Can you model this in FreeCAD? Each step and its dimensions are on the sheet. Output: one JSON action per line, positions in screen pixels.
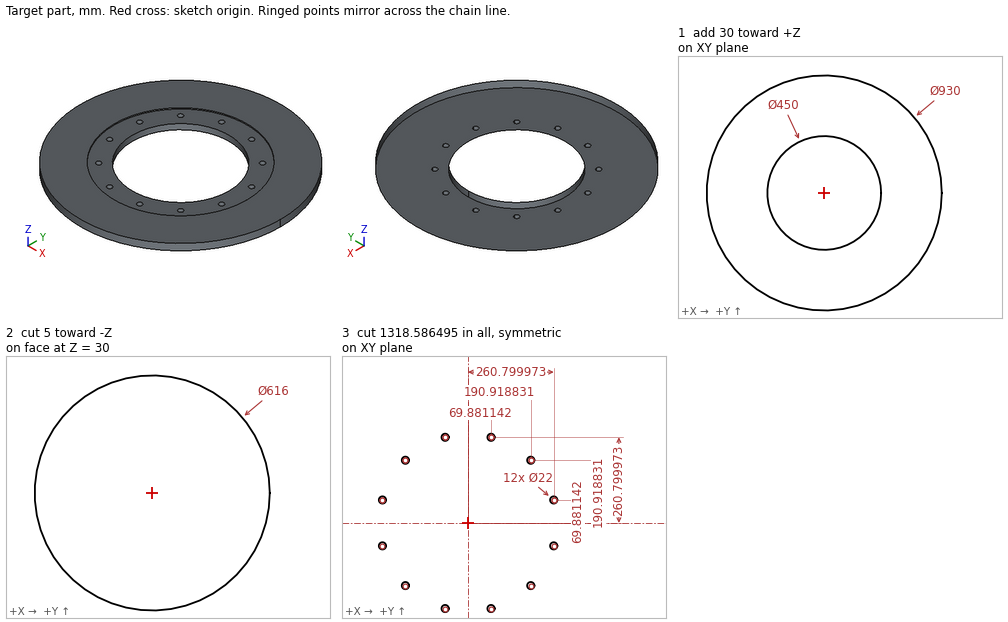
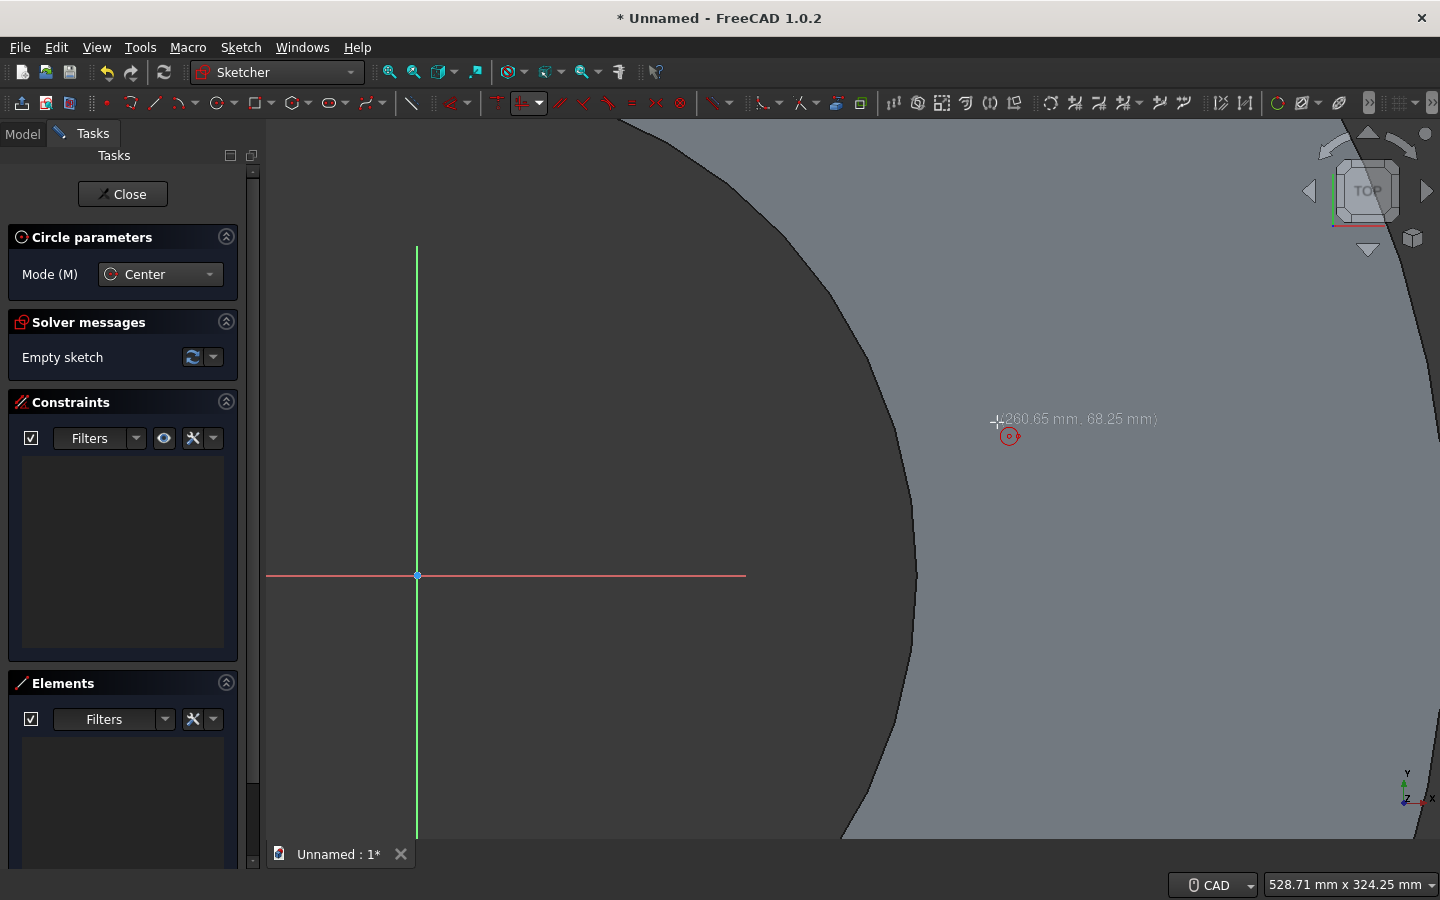
{"action": "left_click", "coordinate": [996, 420]}
{"action": "mouse_move", "coordinate": [1014, 403]}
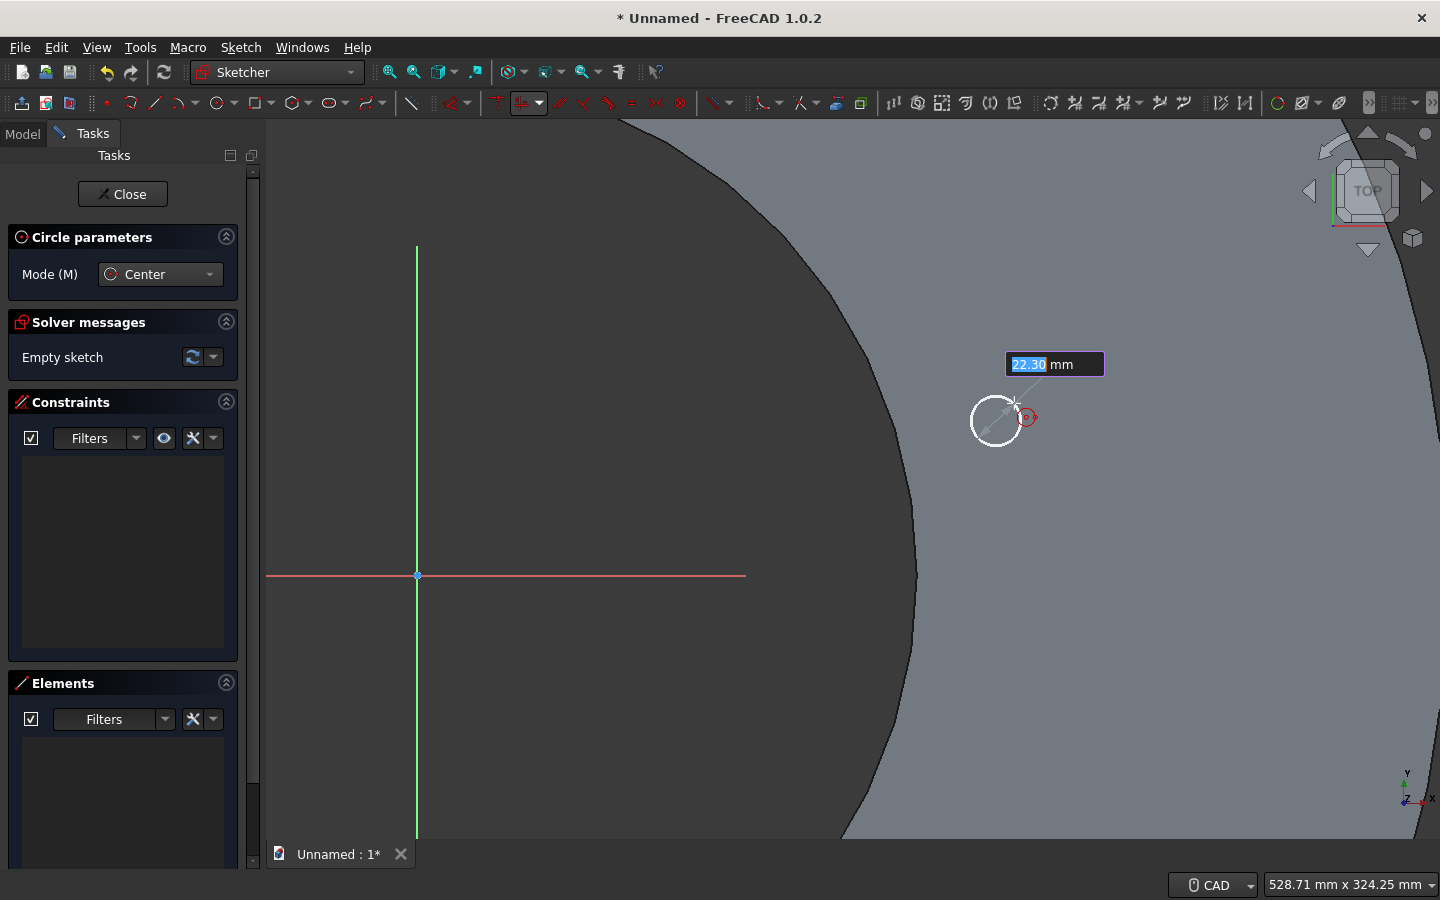
{"action": "type", "text": "22"}
{"action": "key", "text": "Return"}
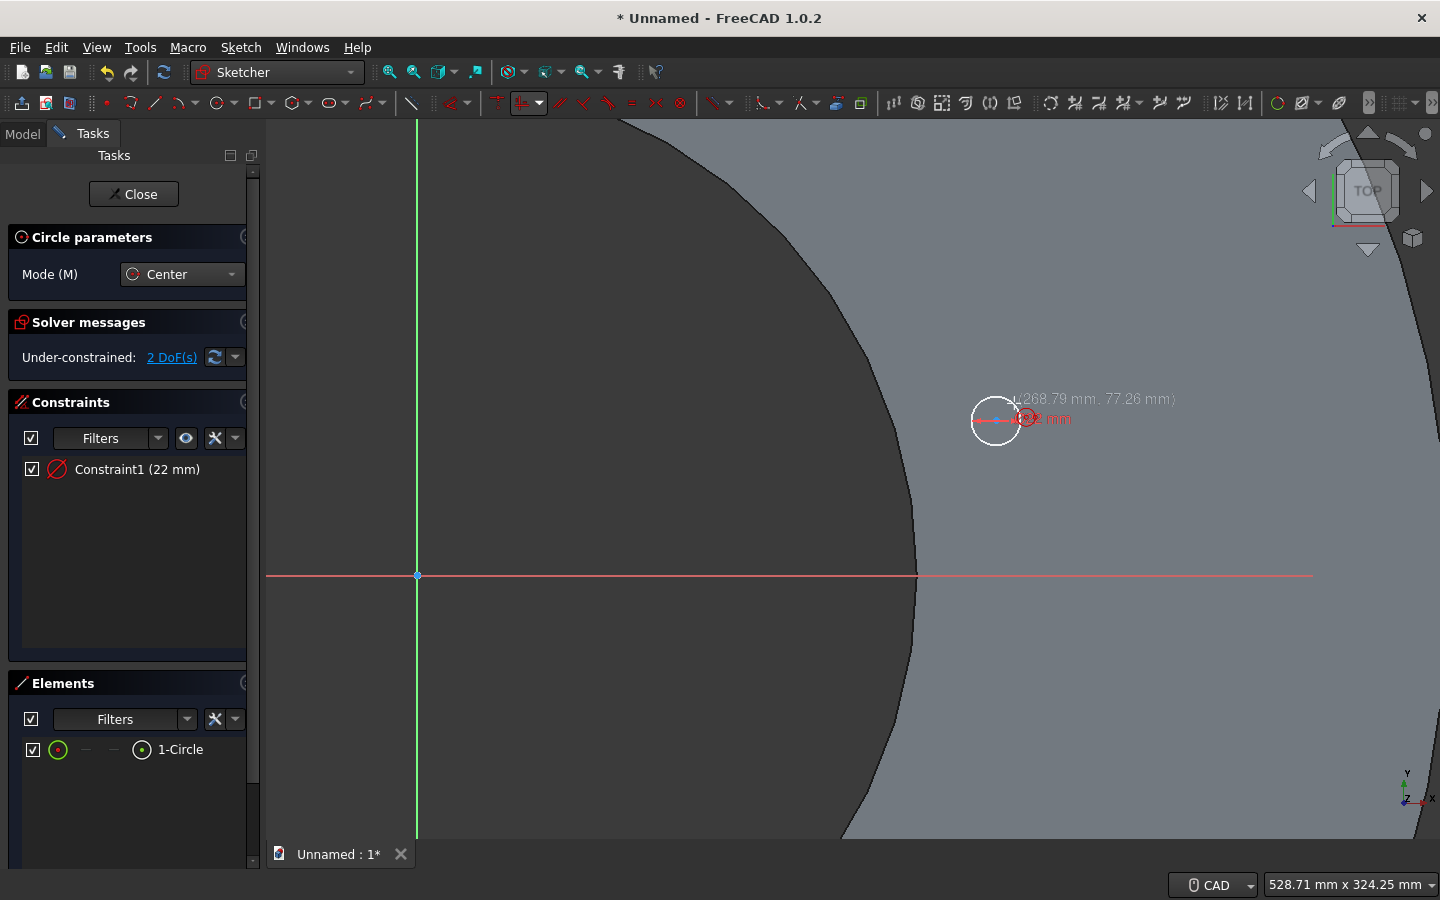
{"action": "left_click", "coordinate": [841, 152]}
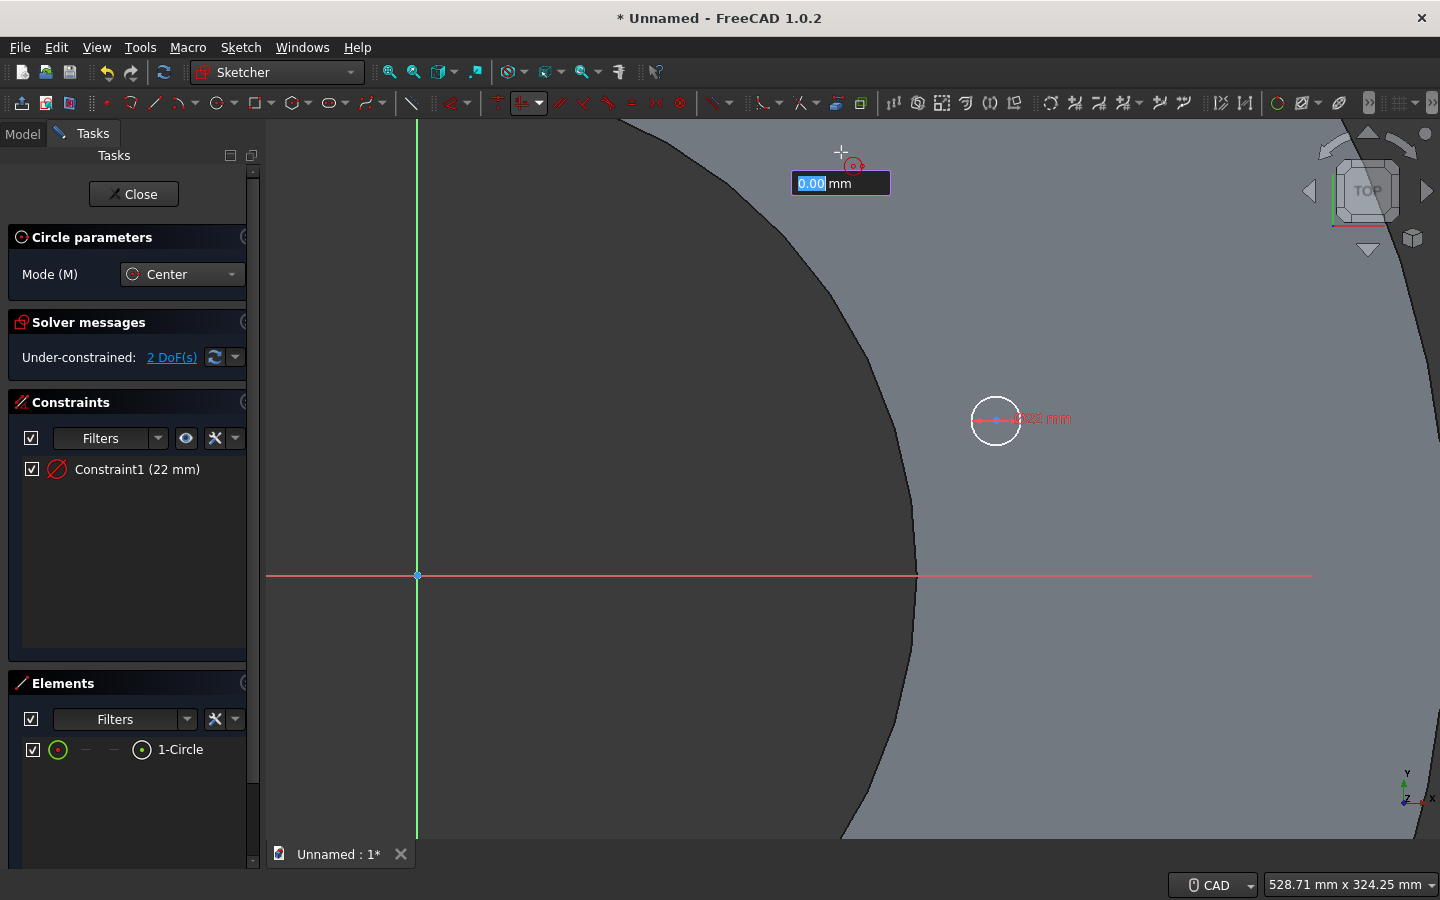
{"action": "scroll", "coordinate": [998, 423], "scroll_direction": "down", "scroll_amount": 5}
{"action": "mouse_move", "coordinate": [947, 317]}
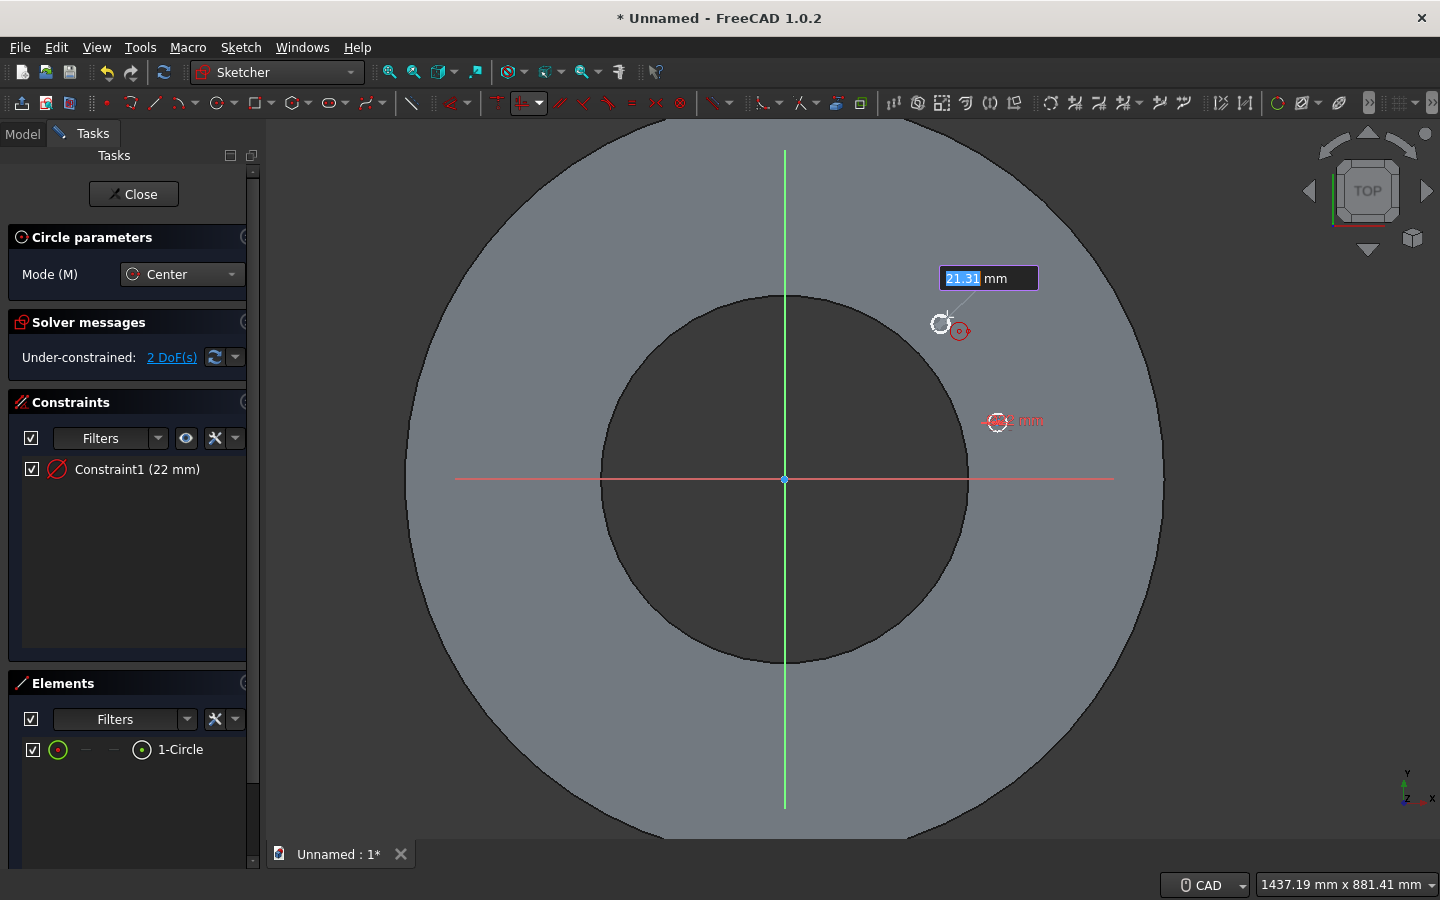
{"action": "type", "text": "22"}
{"action": "key", "text": "Return"}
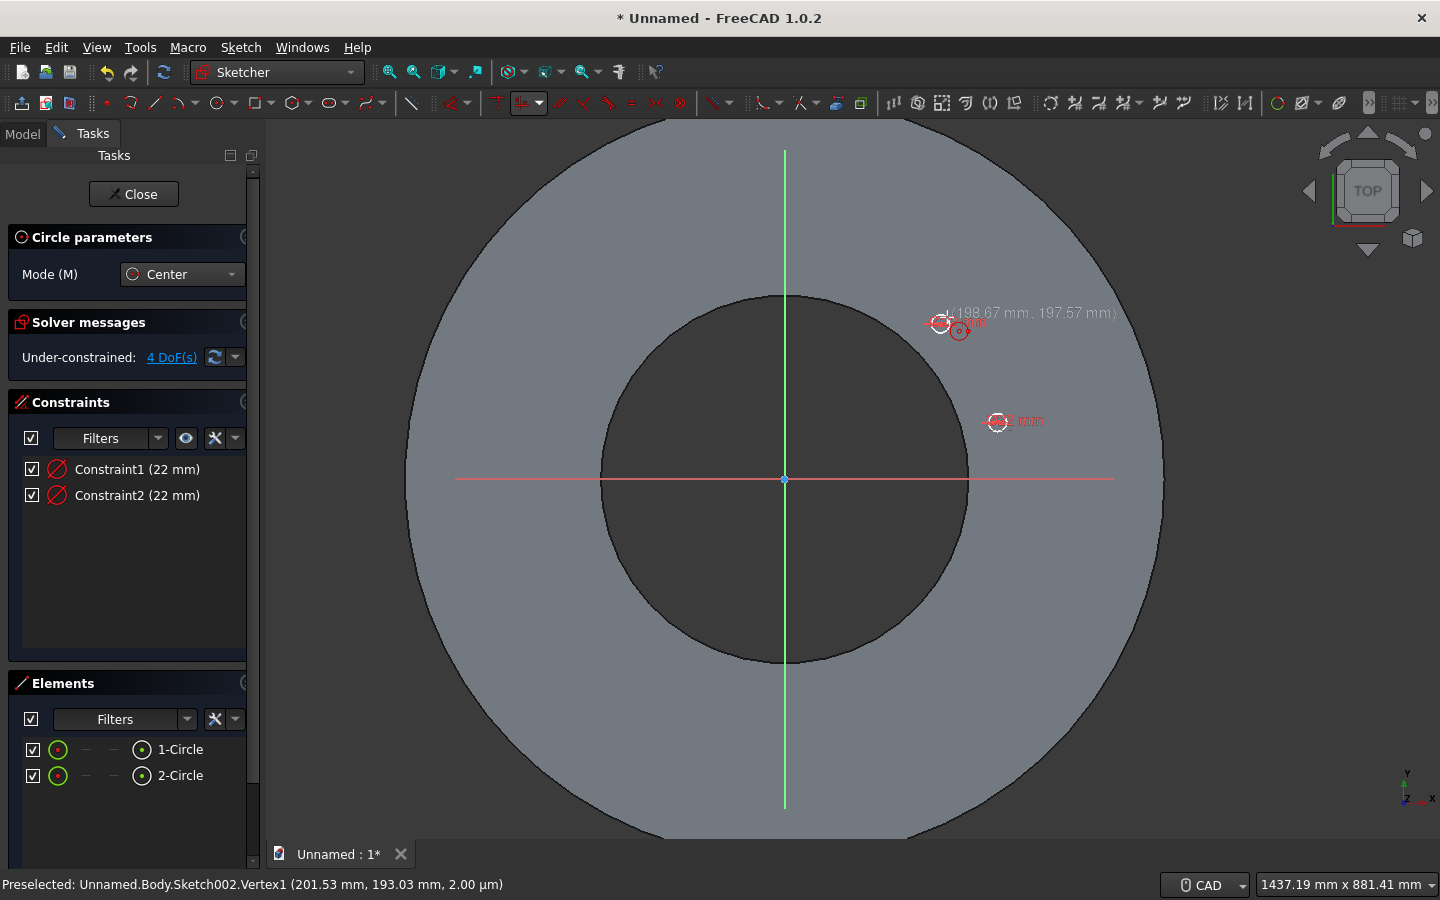
{"action": "scroll", "coordinate": [842, 266], "scroll_direction": "up", "scroll_amount": 5}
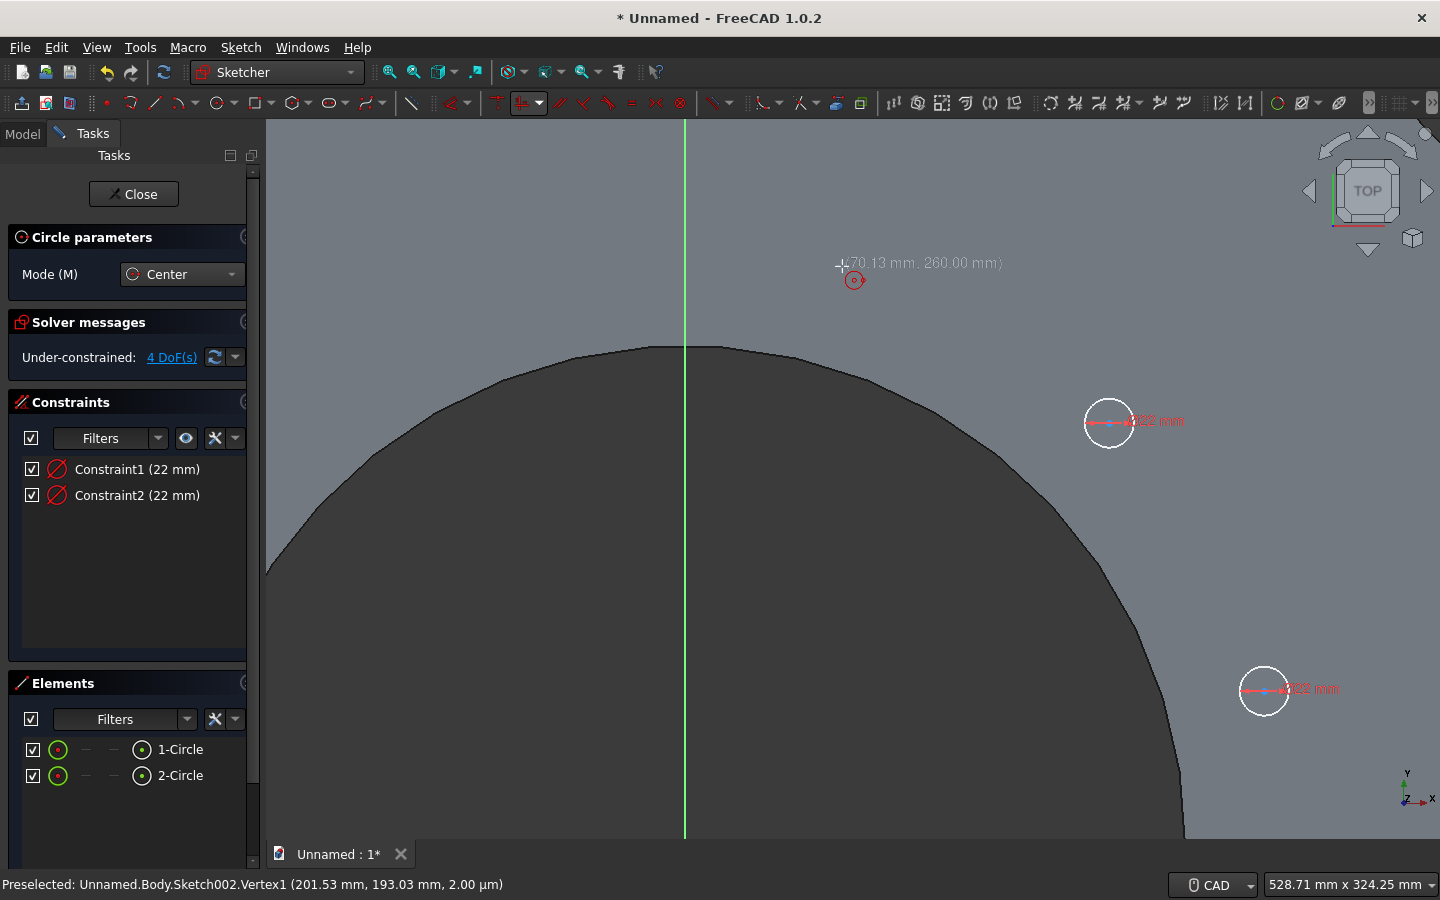
{"action": "left_click", "coordinate": [841, 267]}
{"action": "mouse_move", "coordinate": [858, 249]}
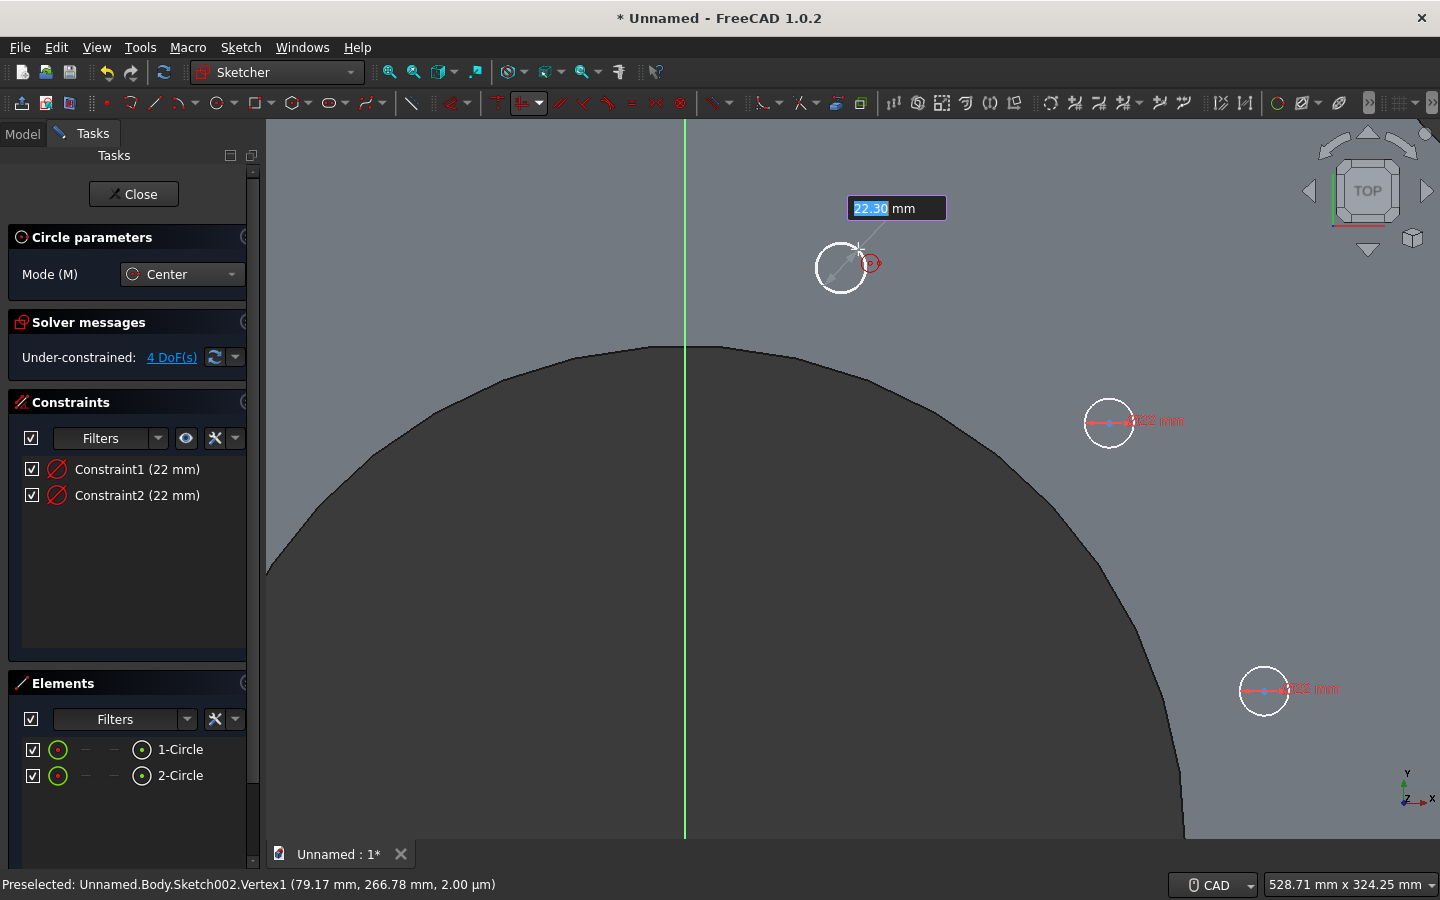
{"action": "type", "text": "22"}
{"action": "key", "text": "Return"}